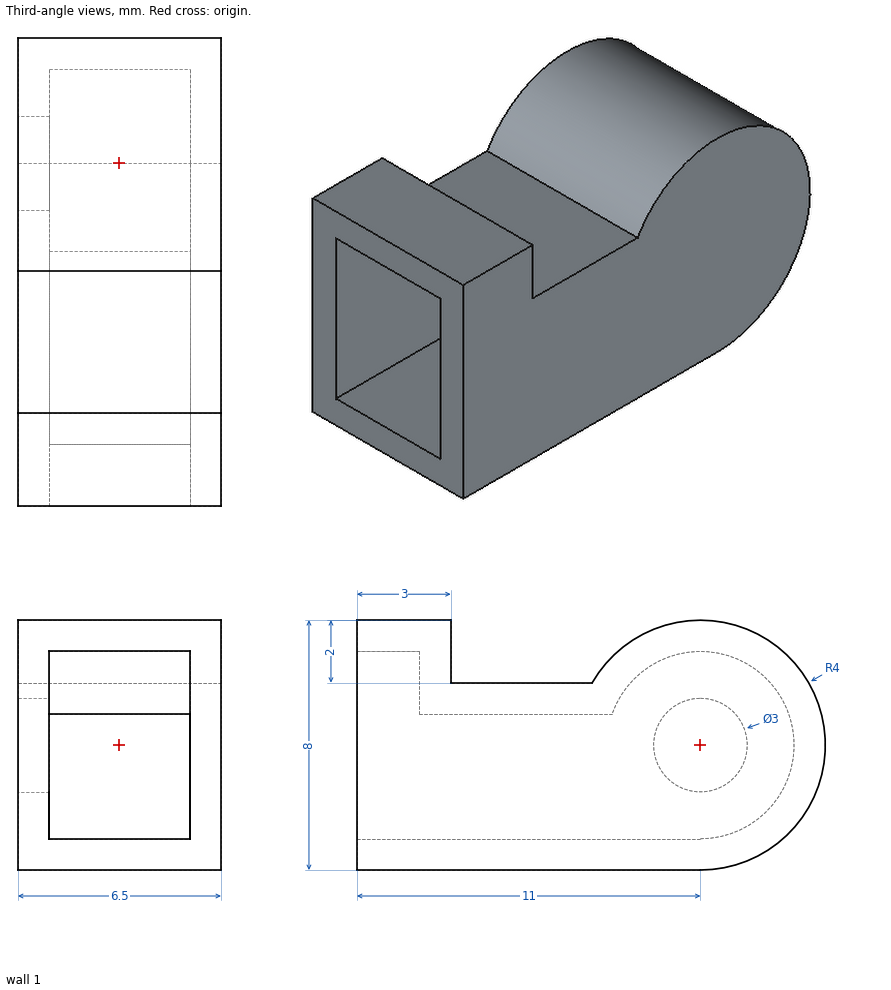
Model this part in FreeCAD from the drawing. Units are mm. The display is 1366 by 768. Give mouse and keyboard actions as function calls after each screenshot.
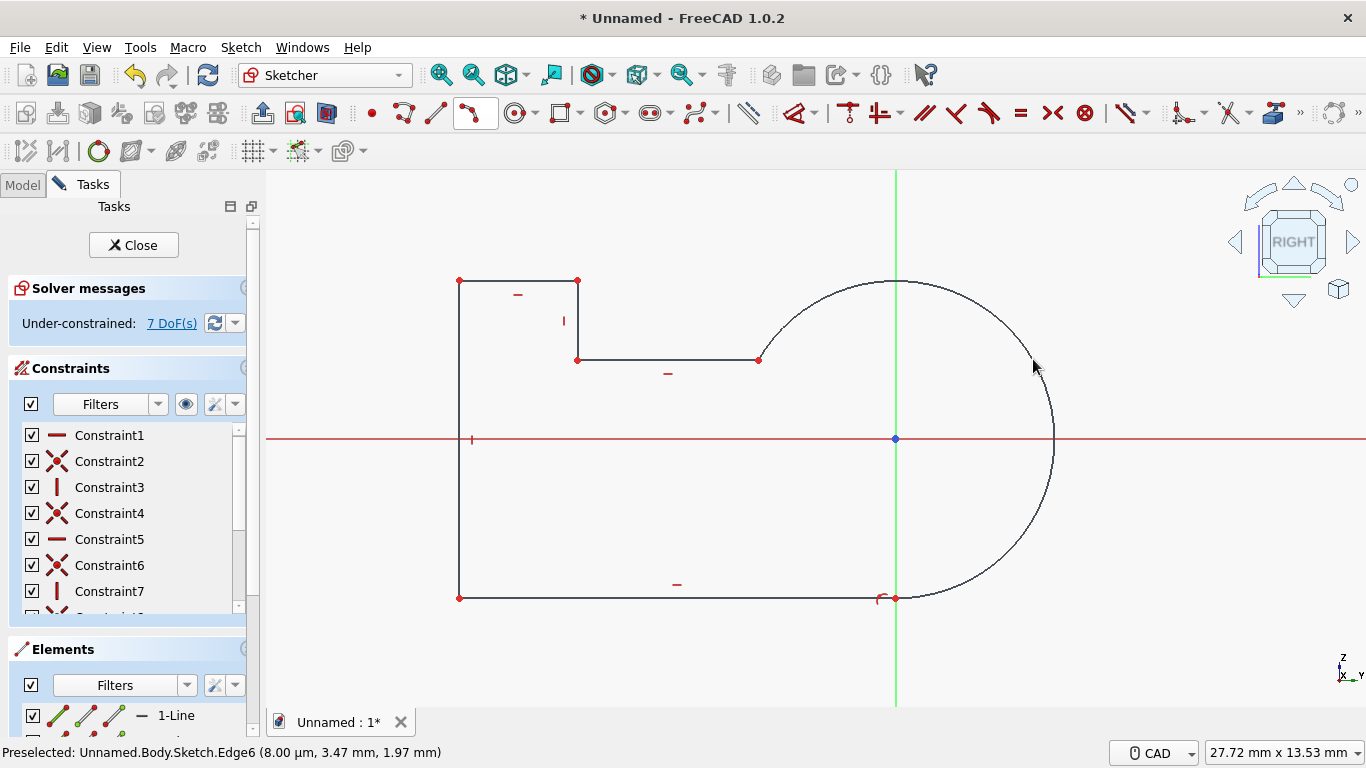
click(590, 598)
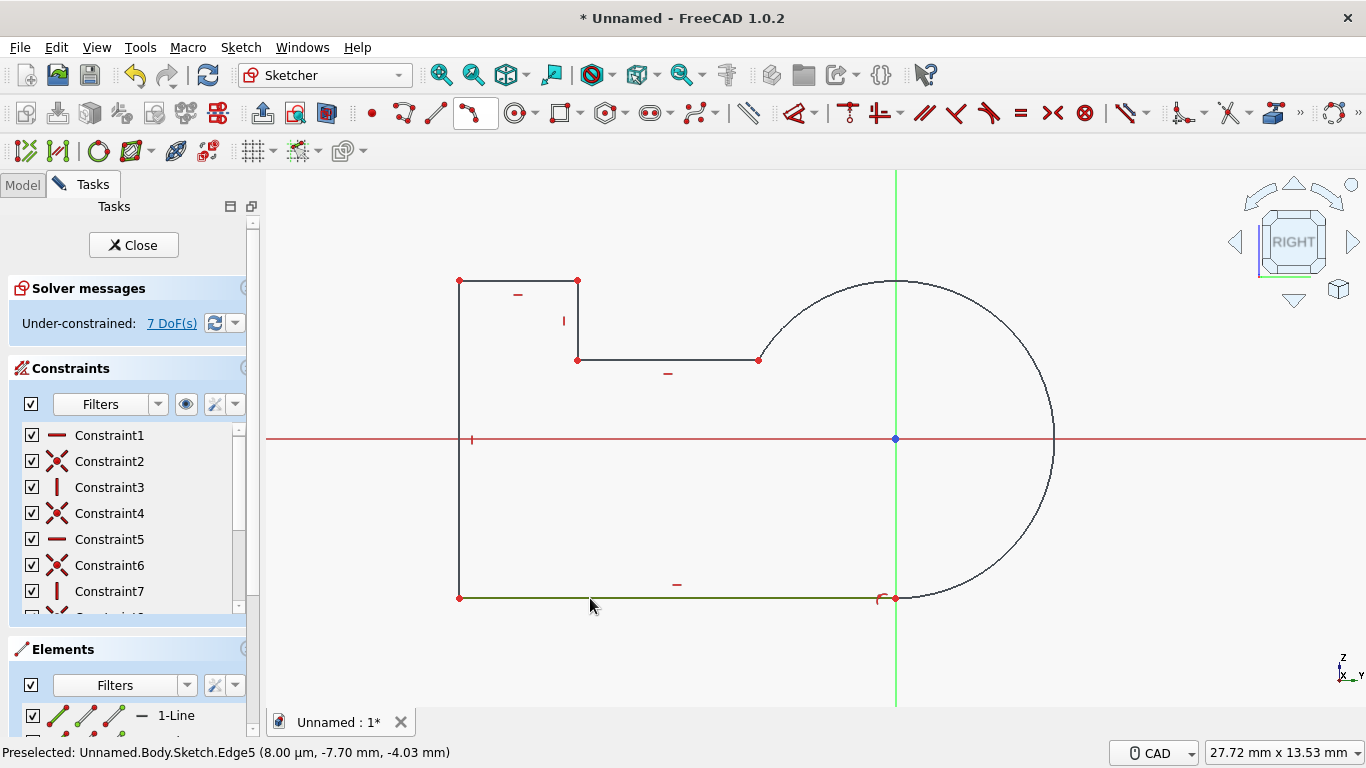
click(1047, 489)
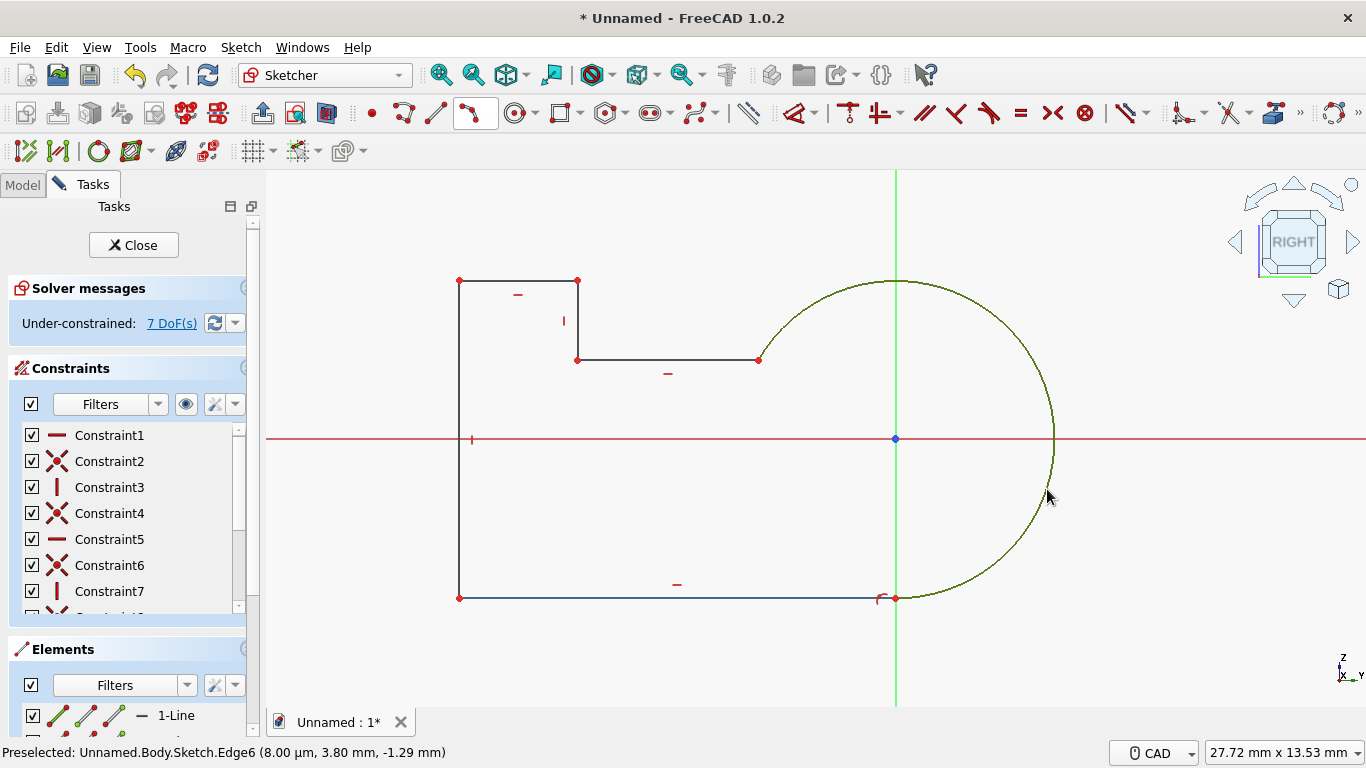
key(t)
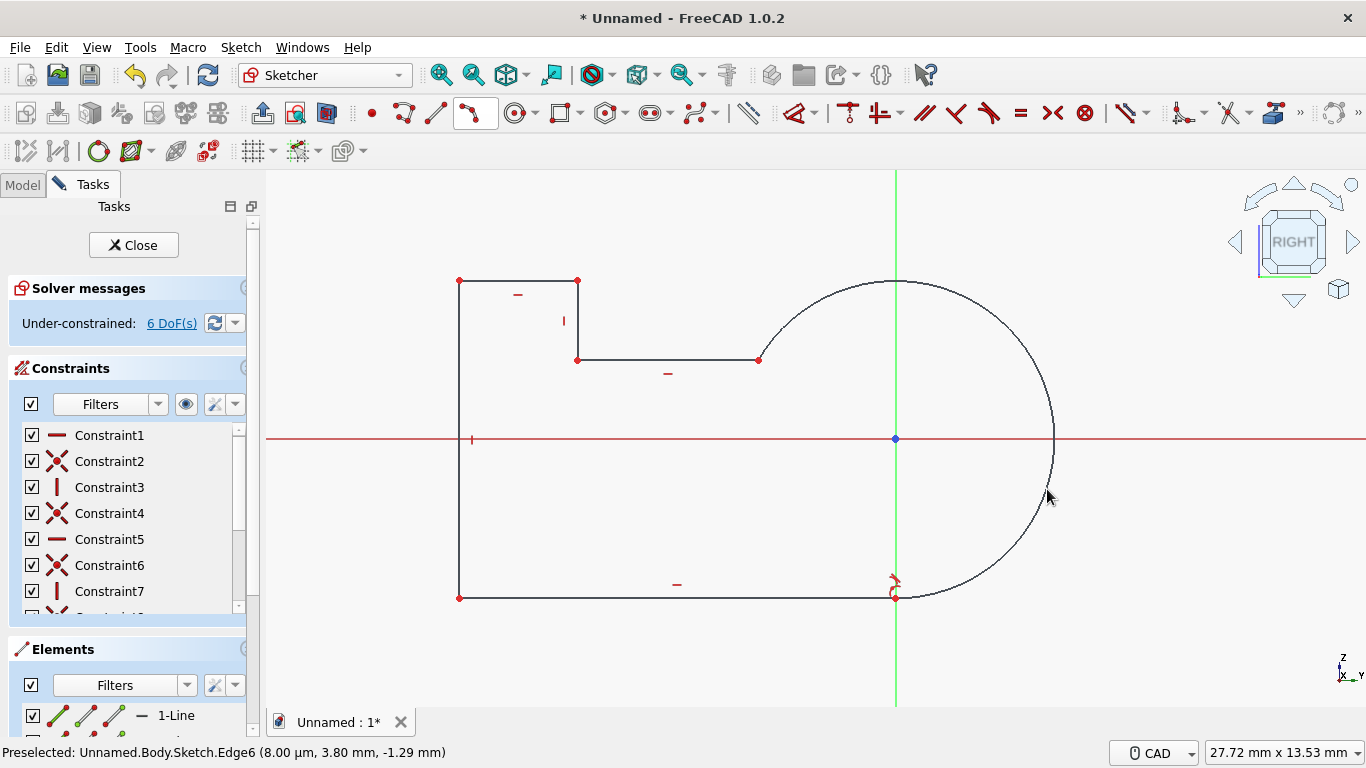
click(896, 440)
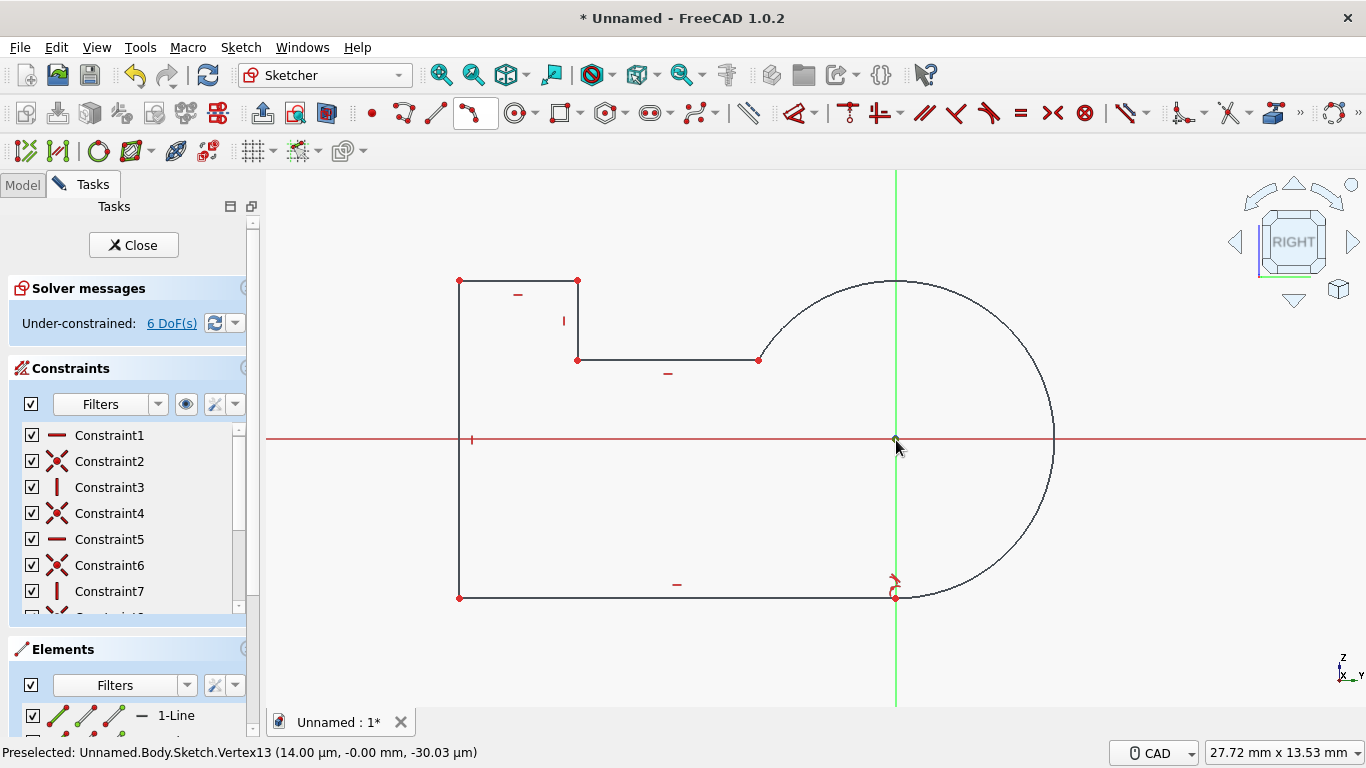
click(359, 438)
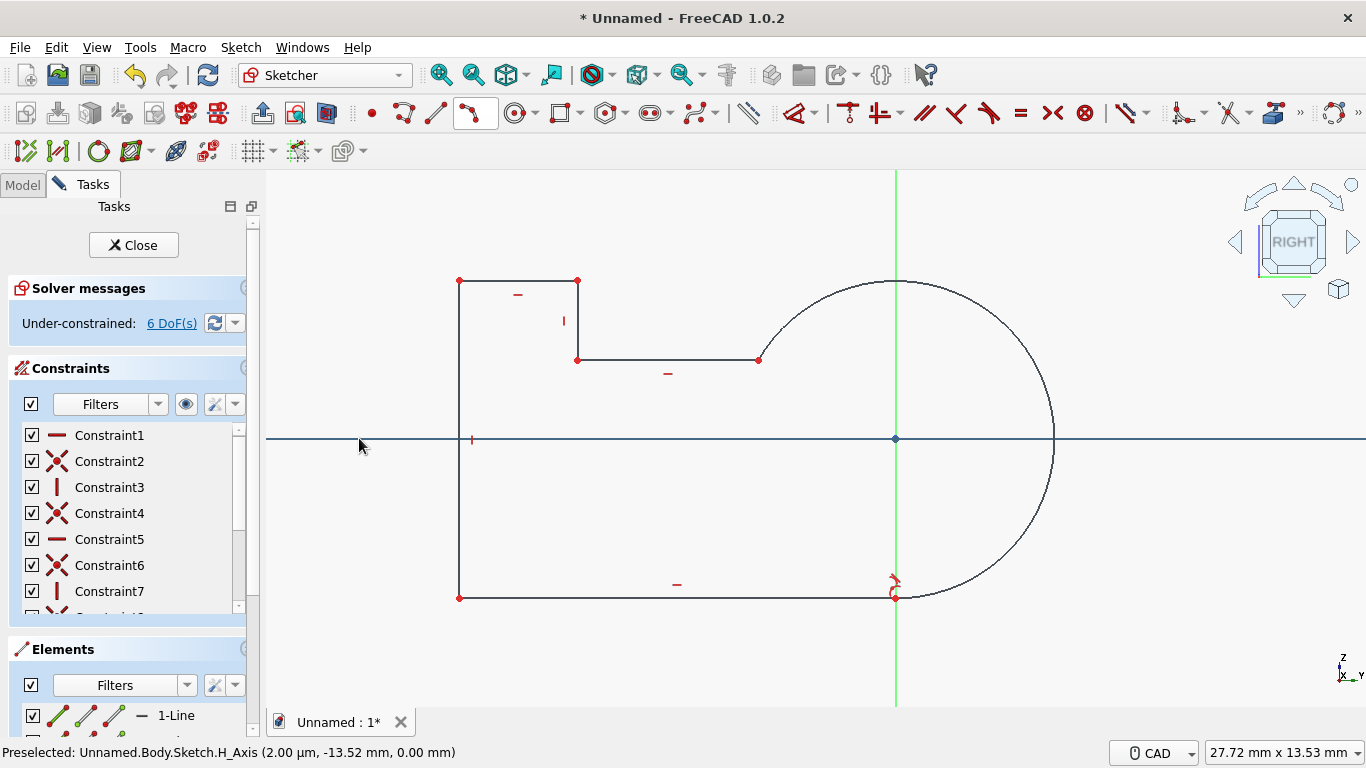
key(c)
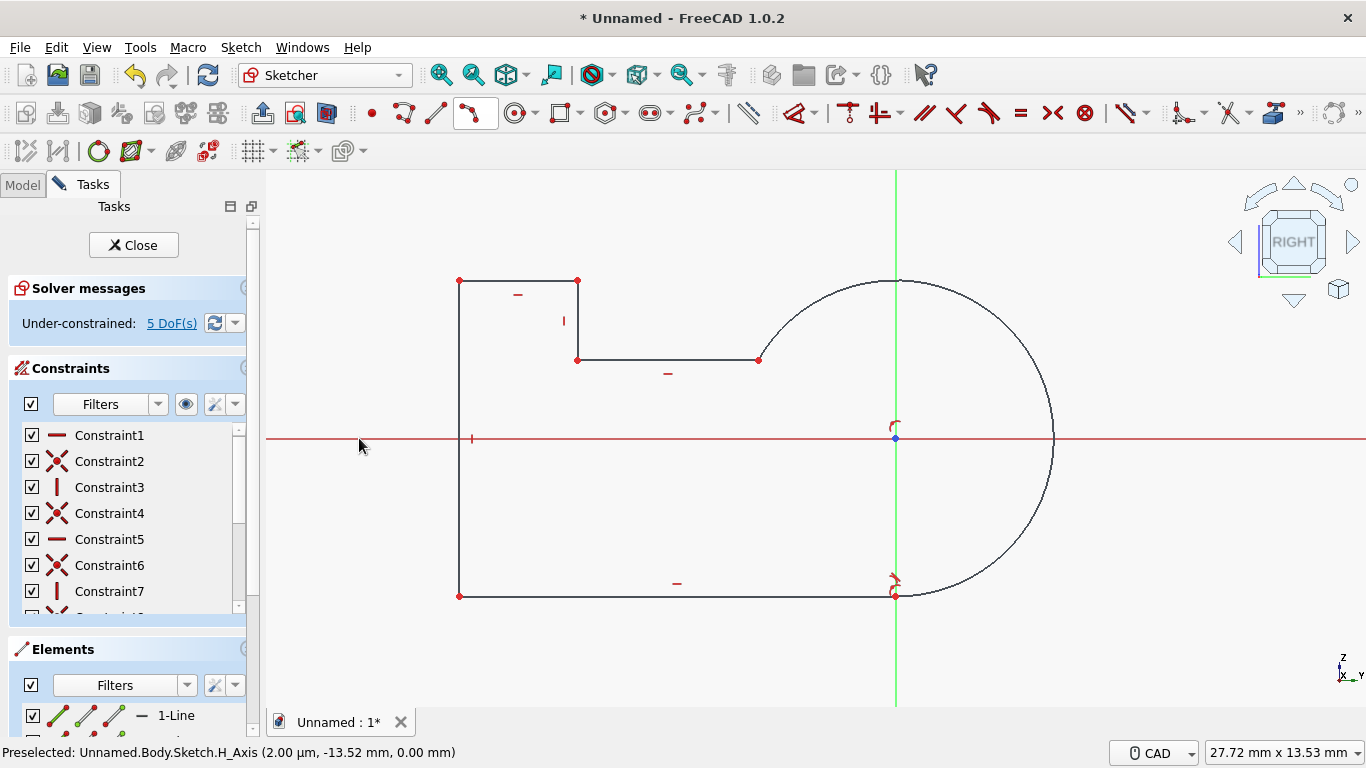
click(1046, 487)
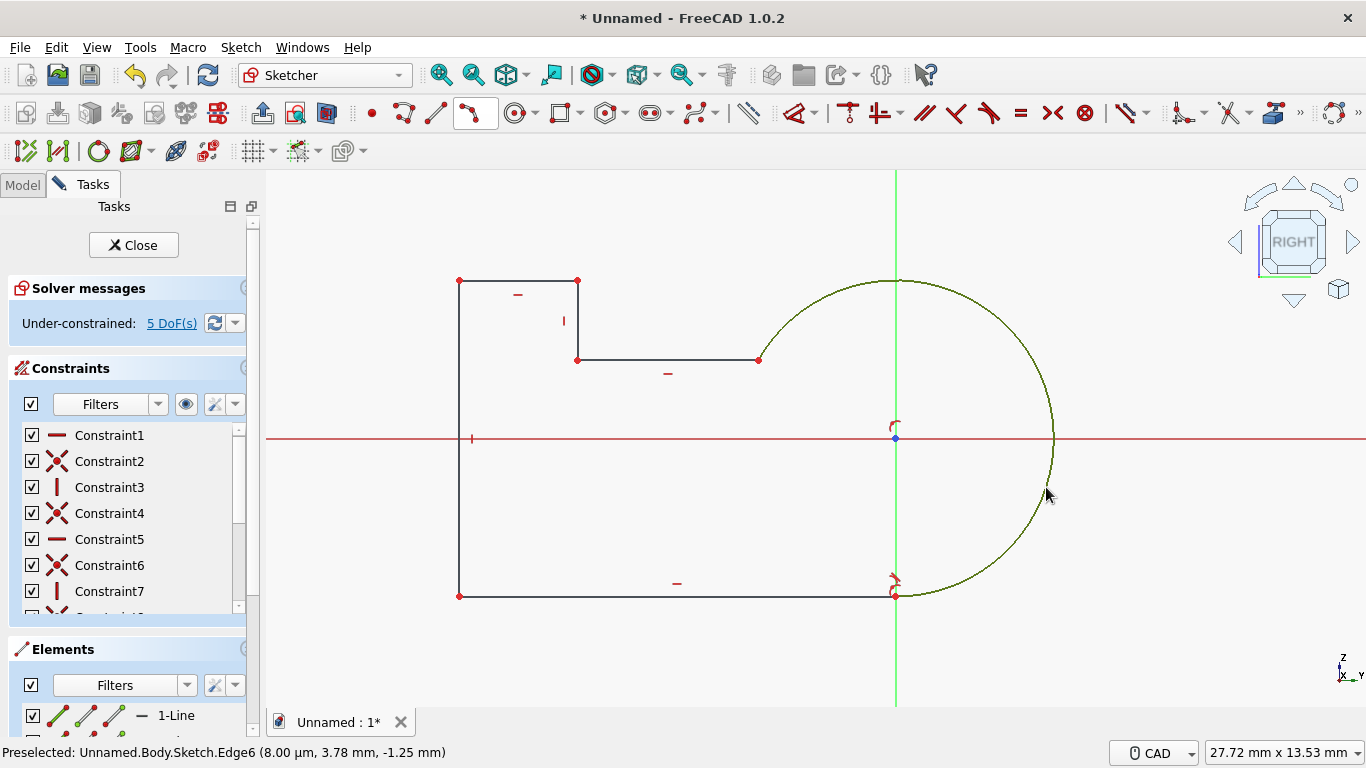
key(k)
key(r)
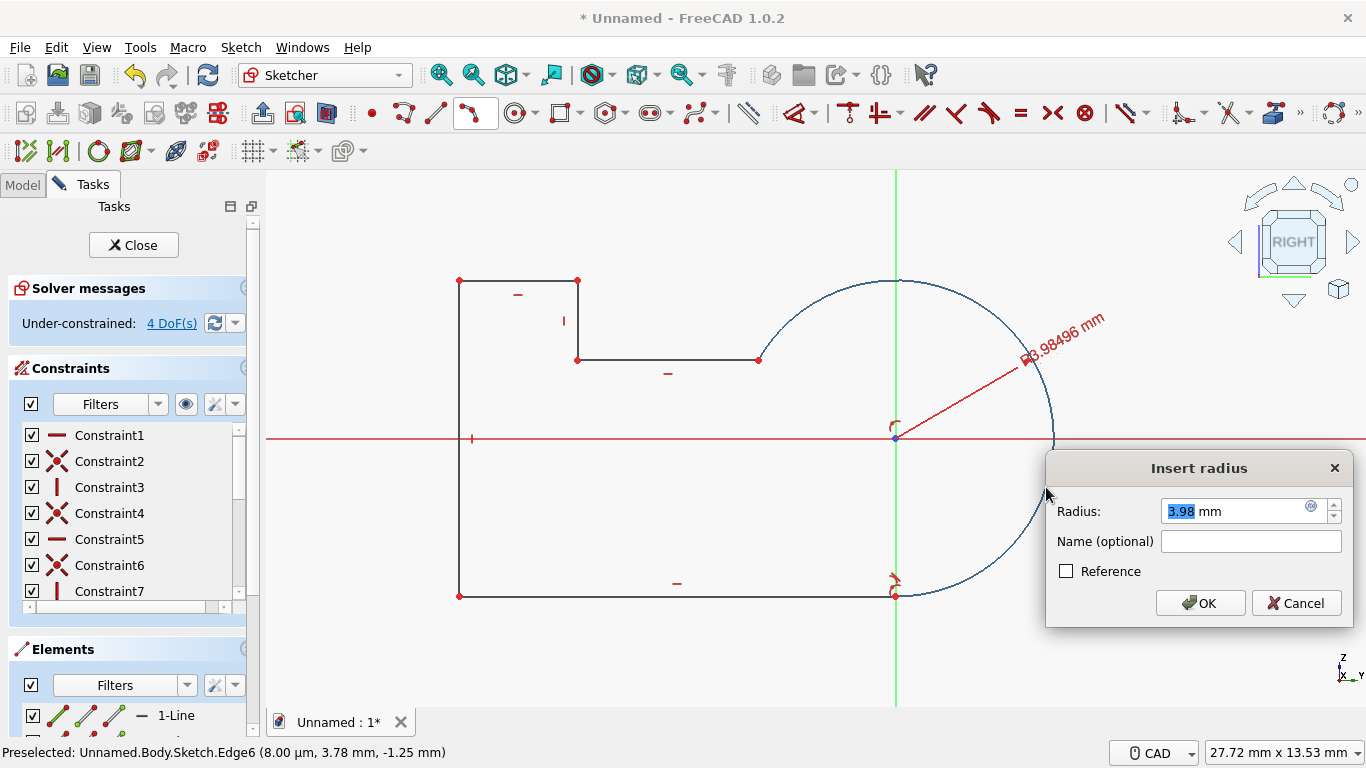
text(4)
key(Return)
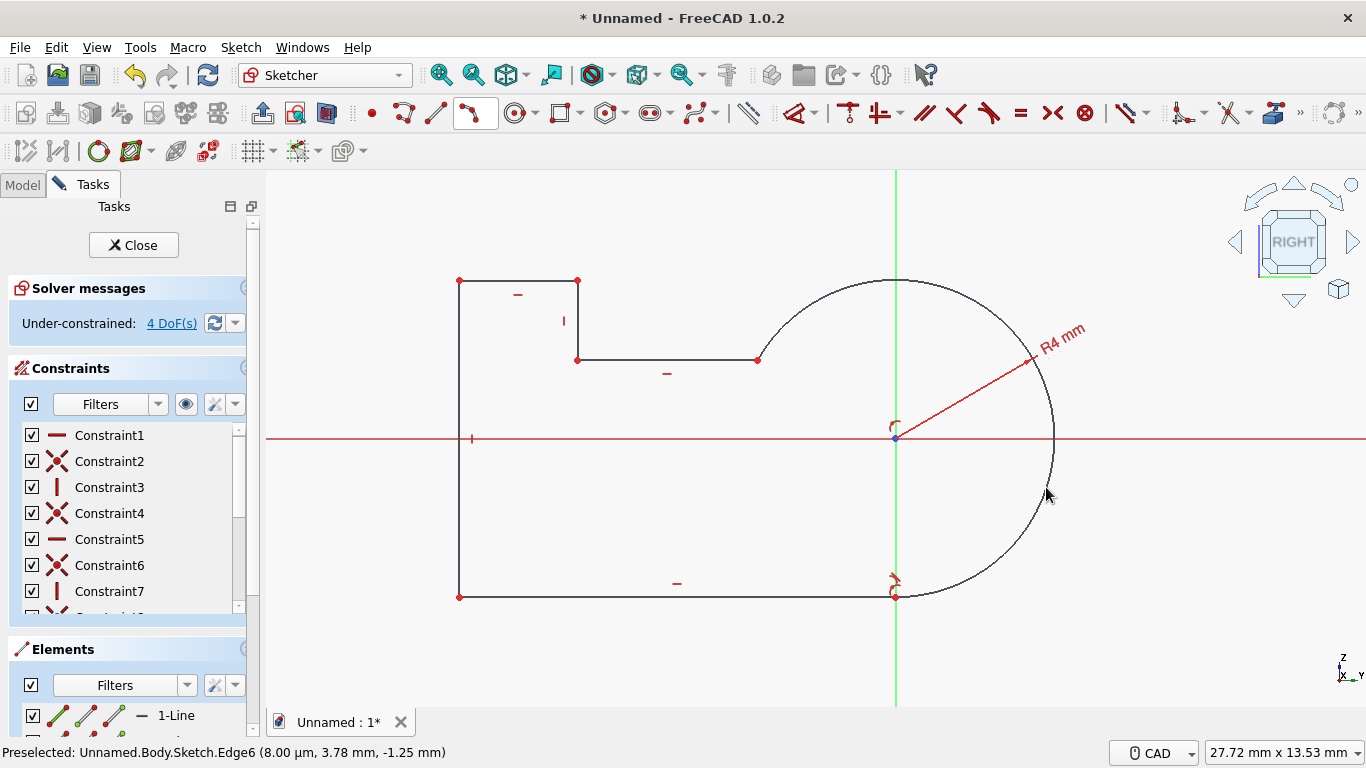
click(578, 336)